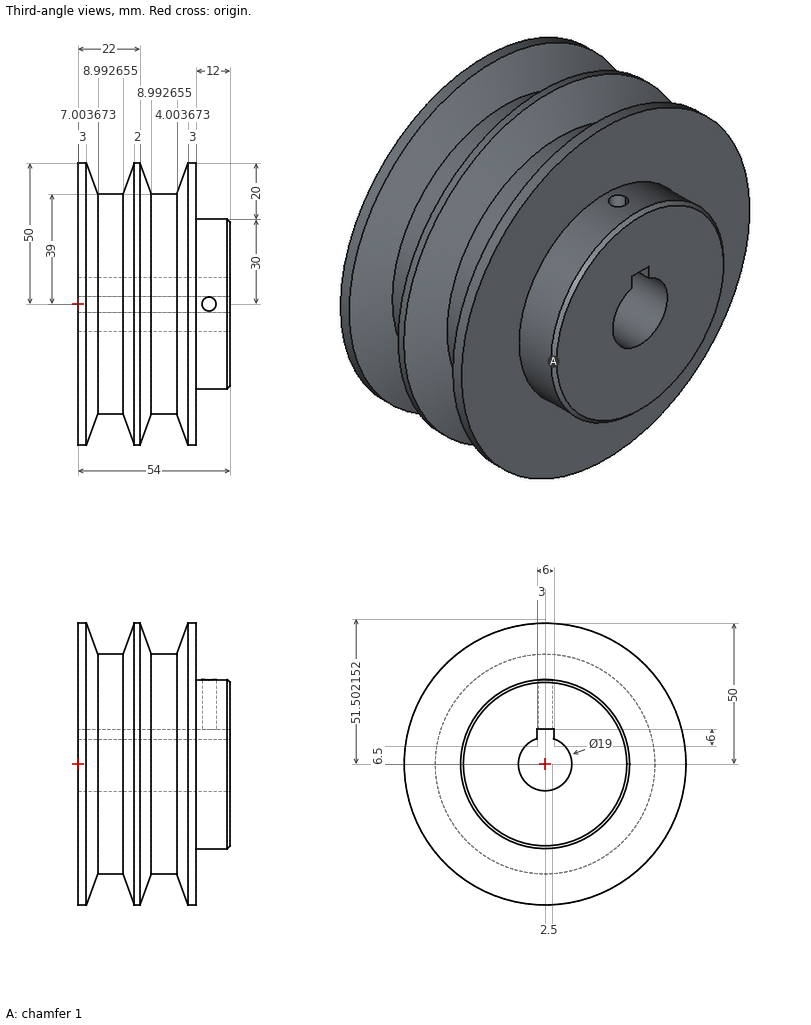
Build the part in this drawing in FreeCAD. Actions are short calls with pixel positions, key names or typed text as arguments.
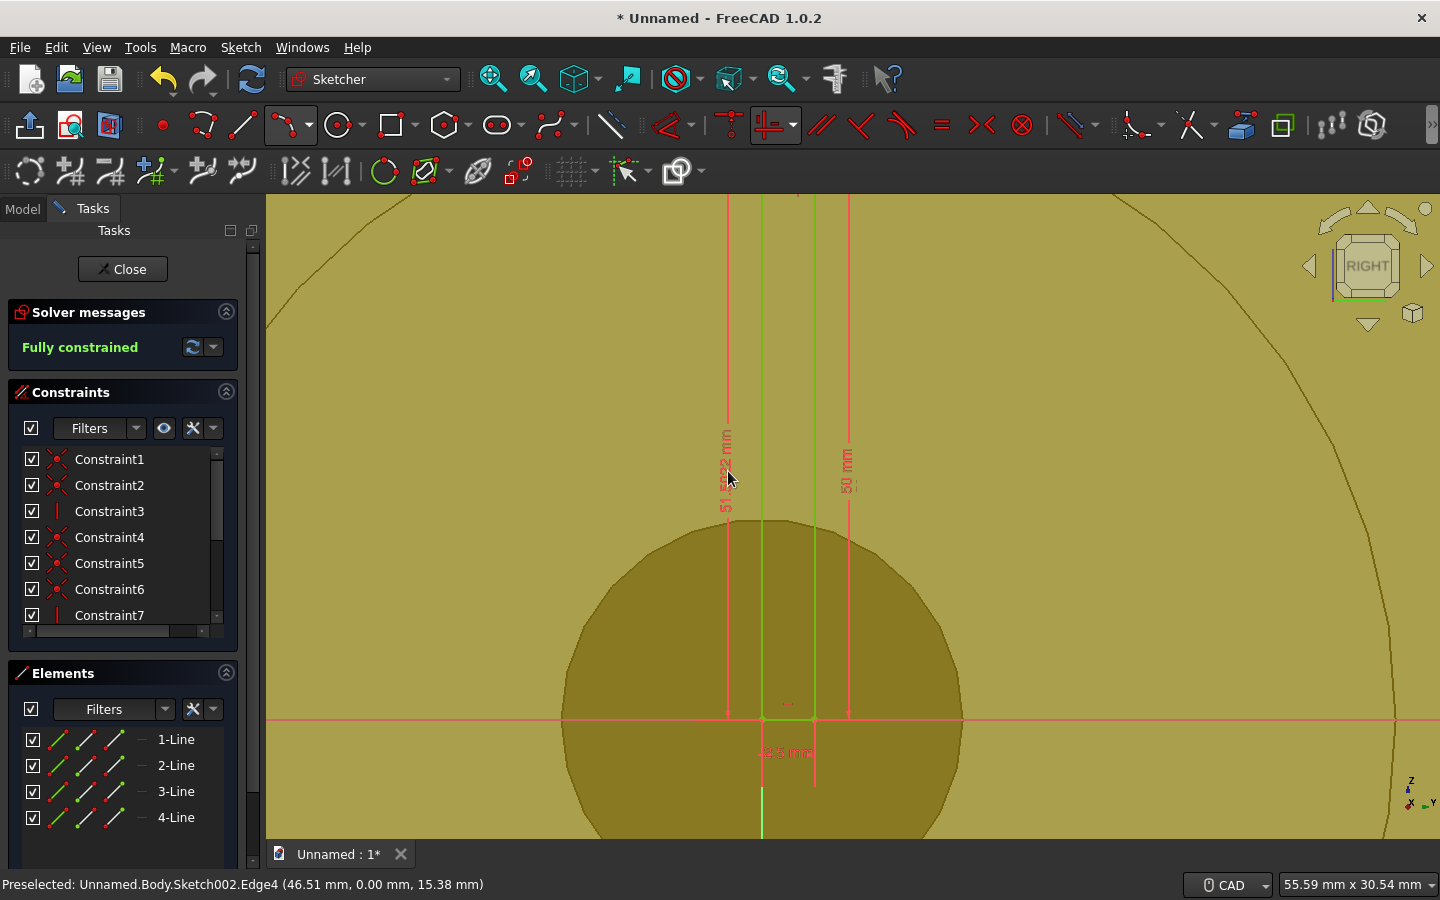
click(123, 269)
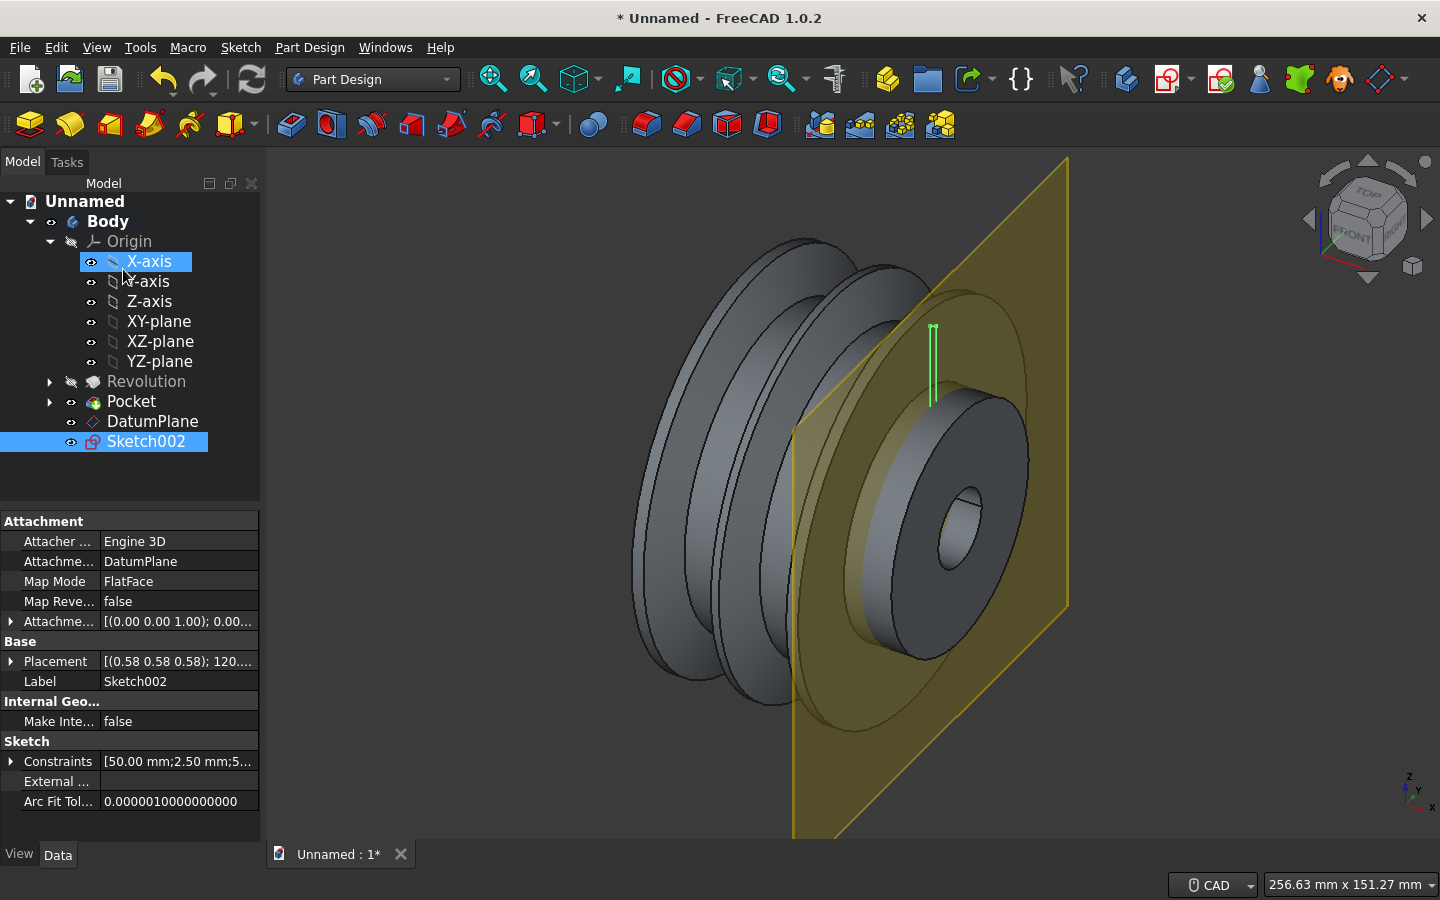
click(372, 124)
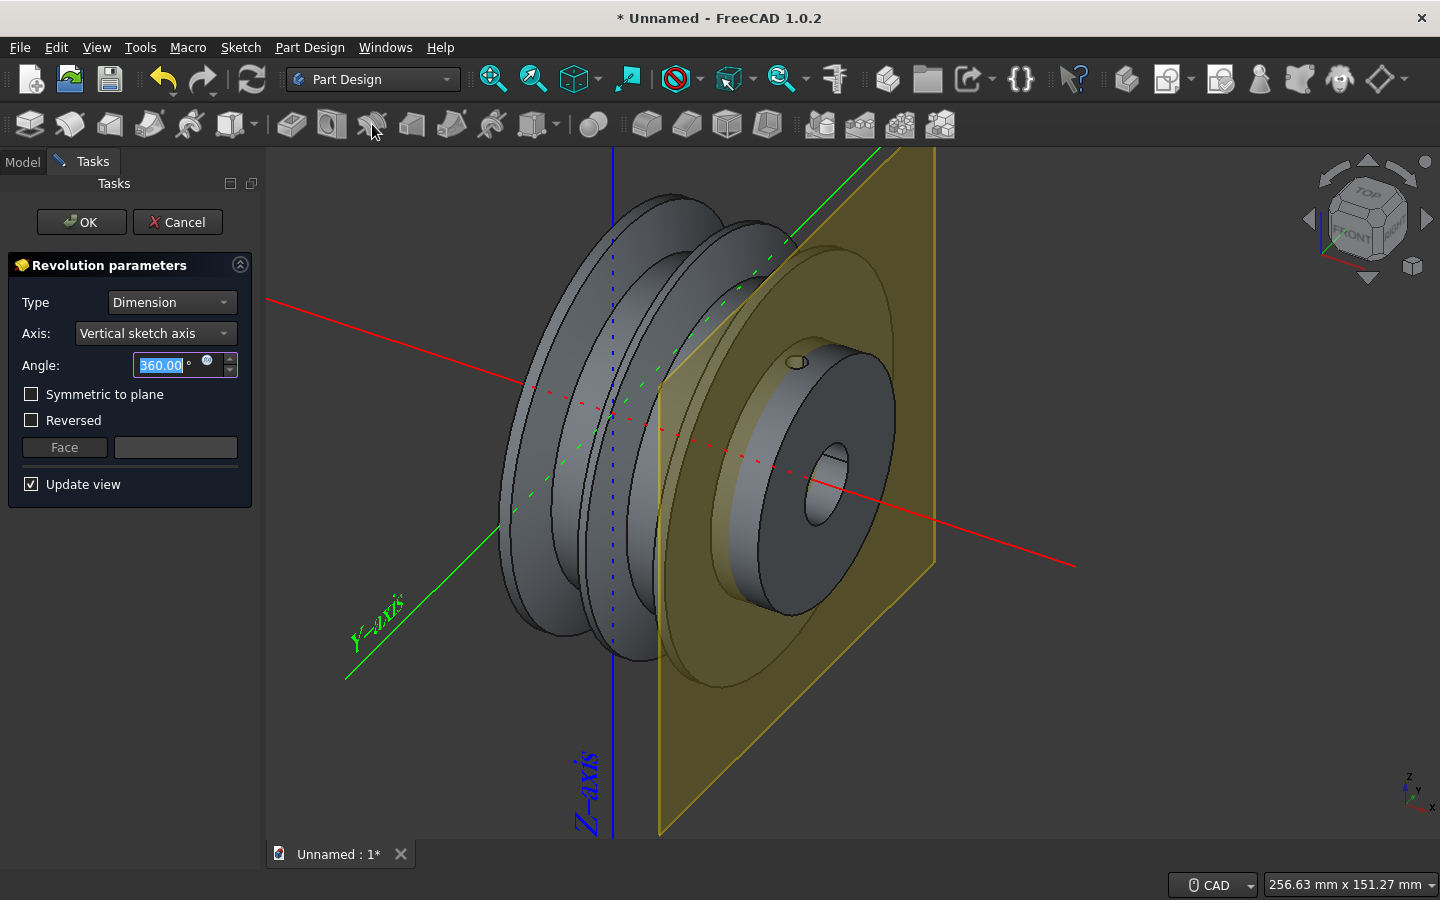
click(82, 222)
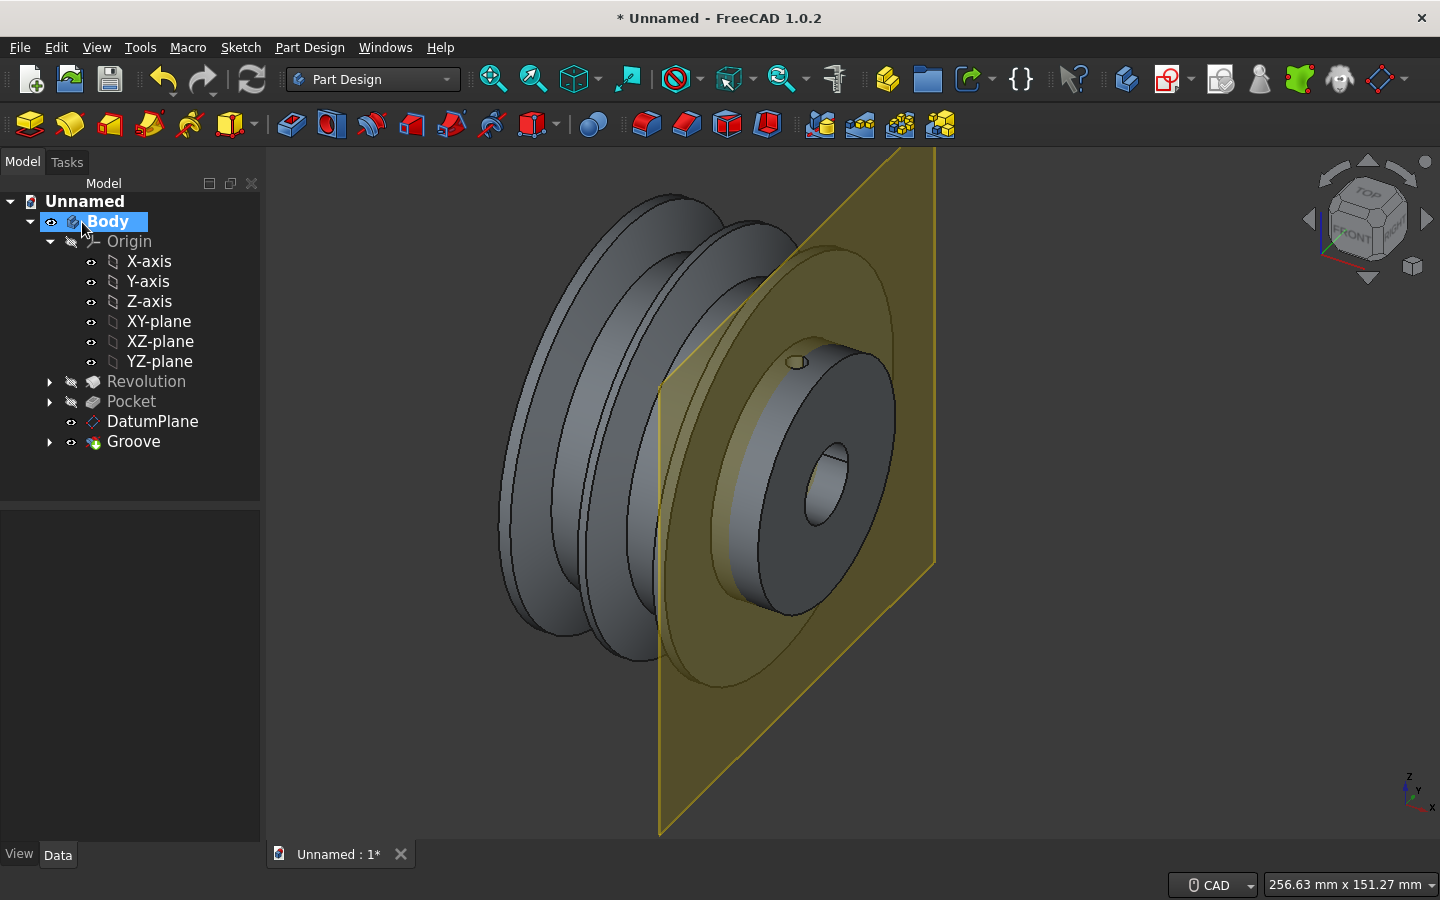
click(116, 422)
key(space)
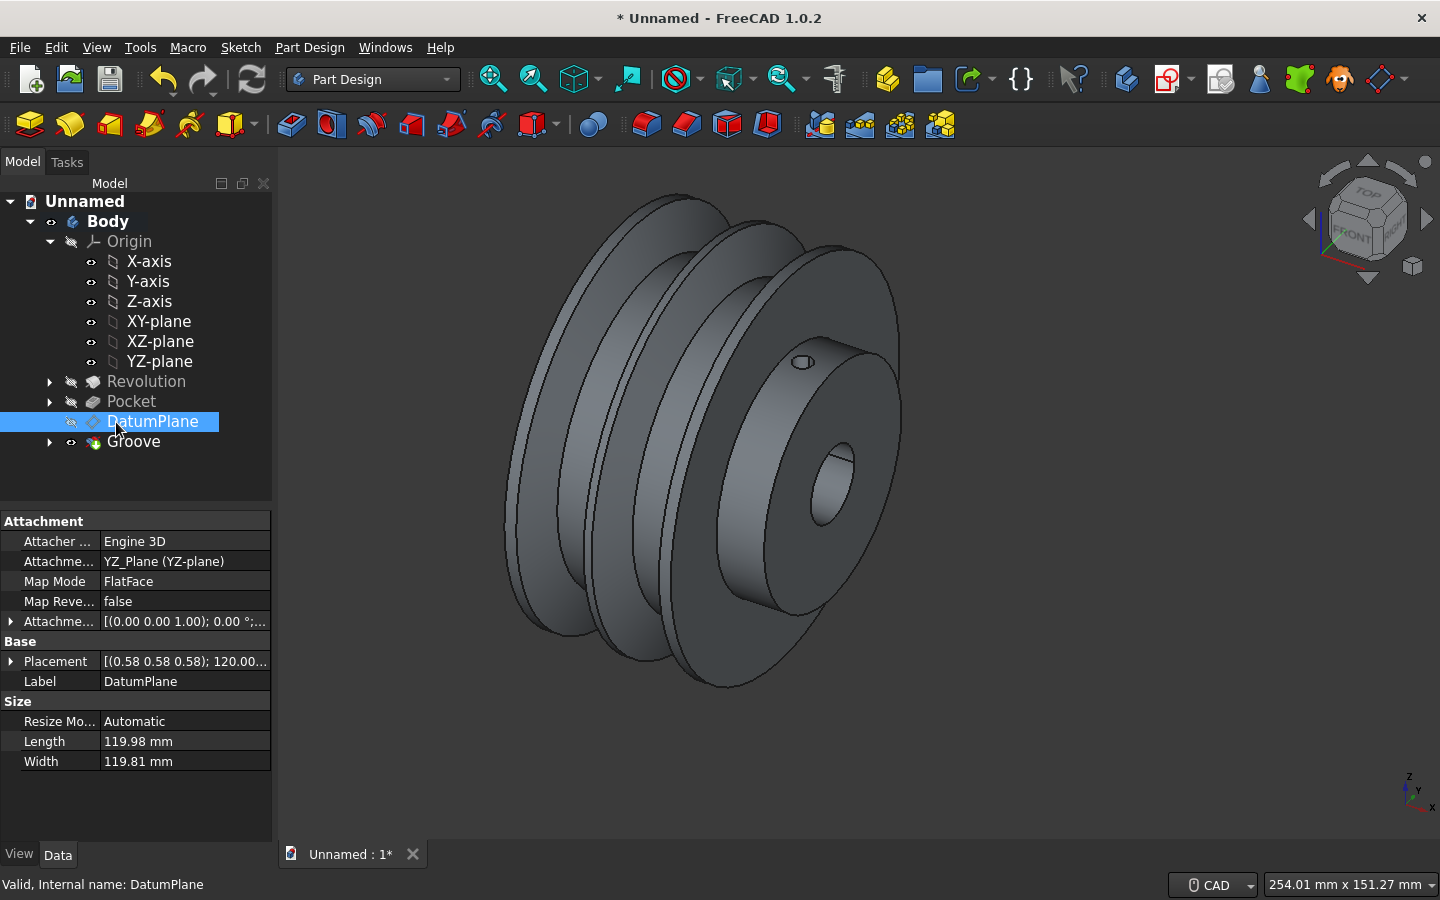
click(494, 80)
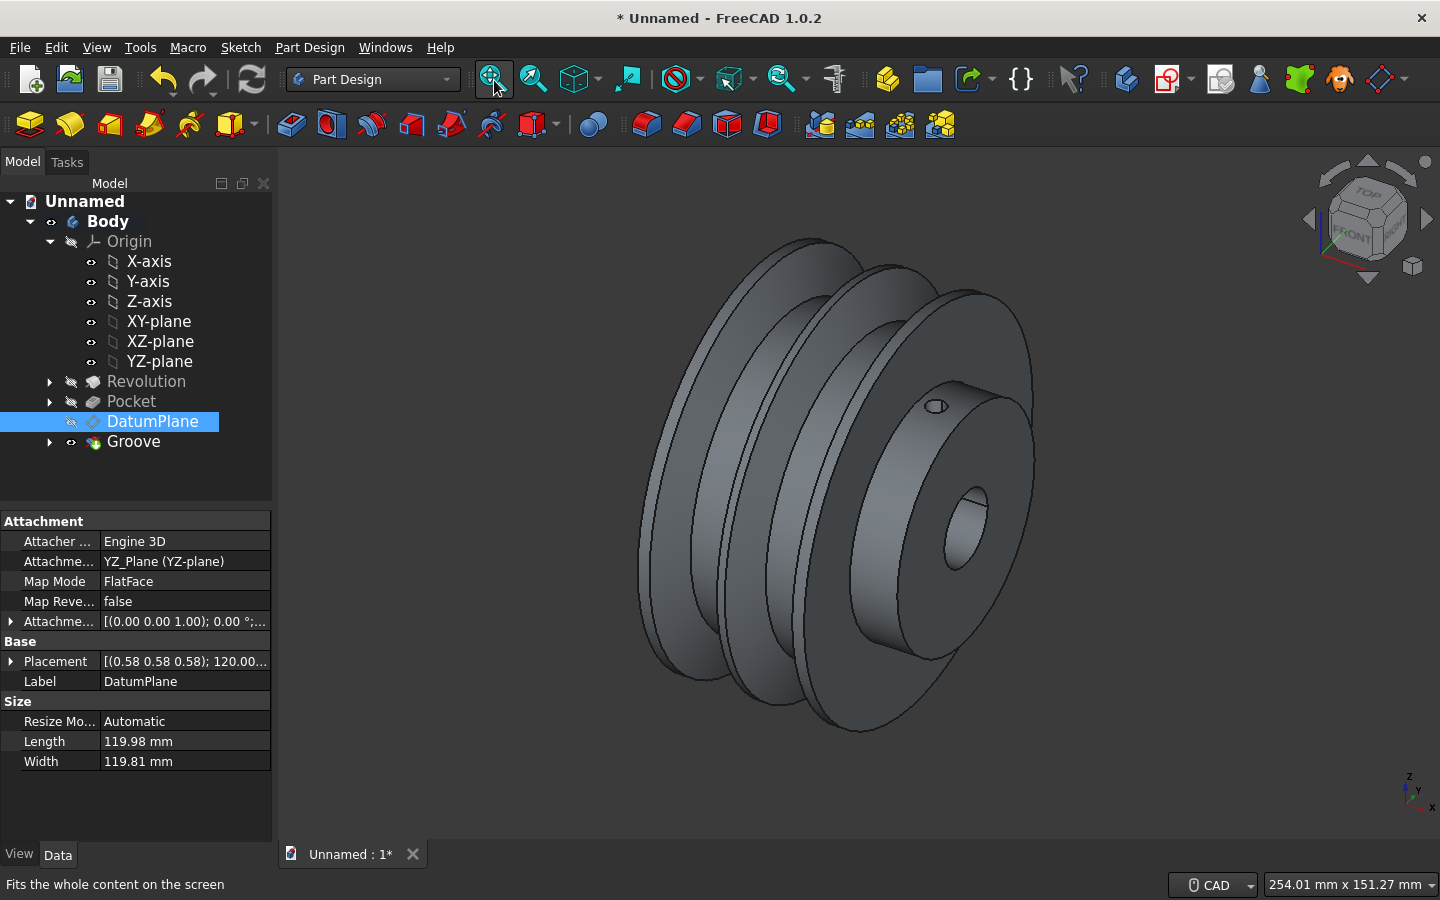
click(897, 596)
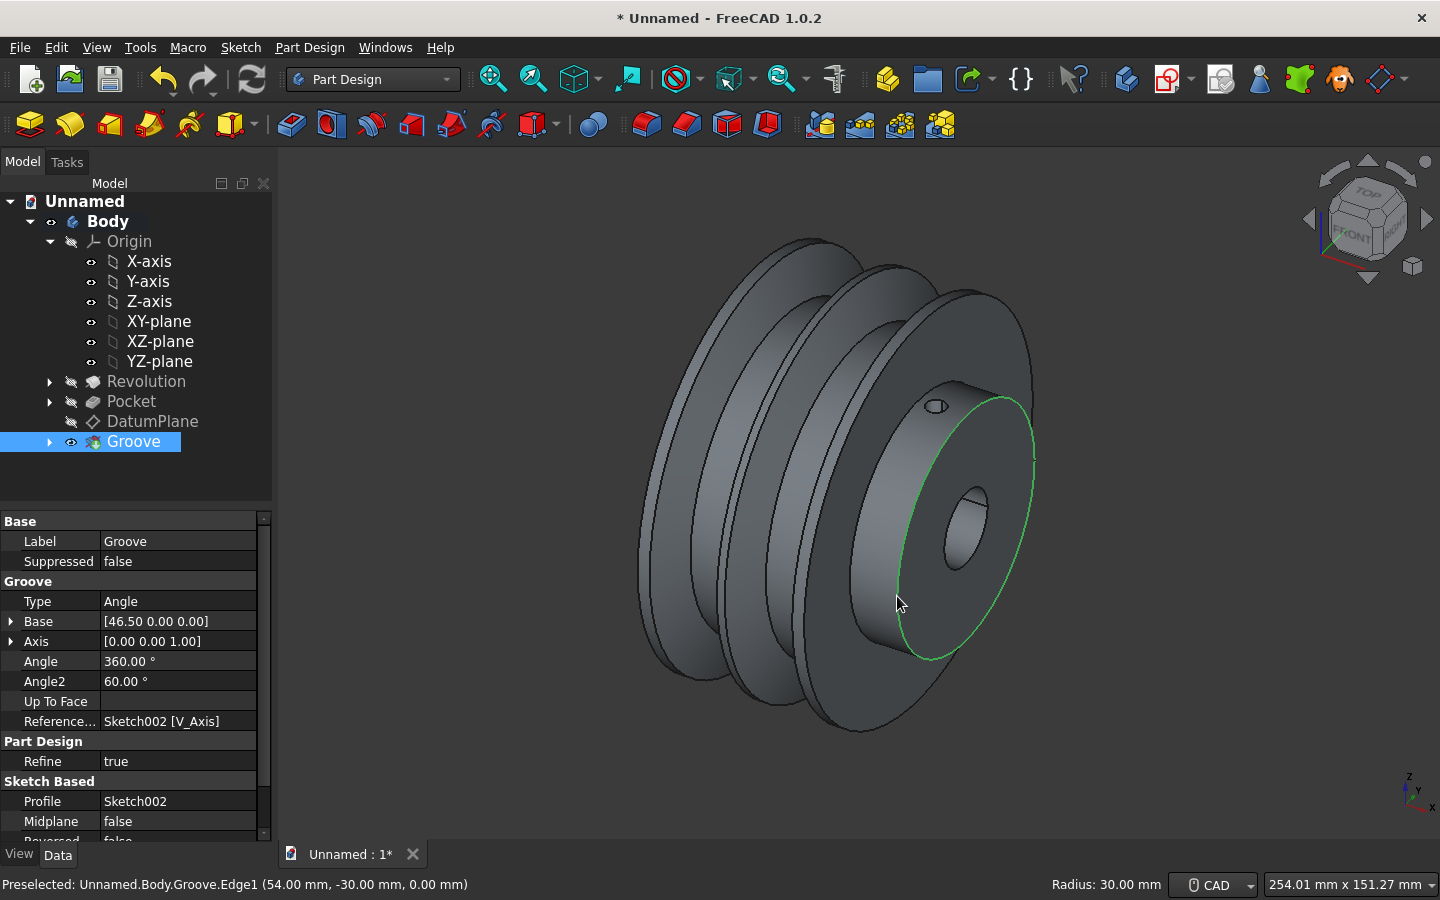
click(688, 124)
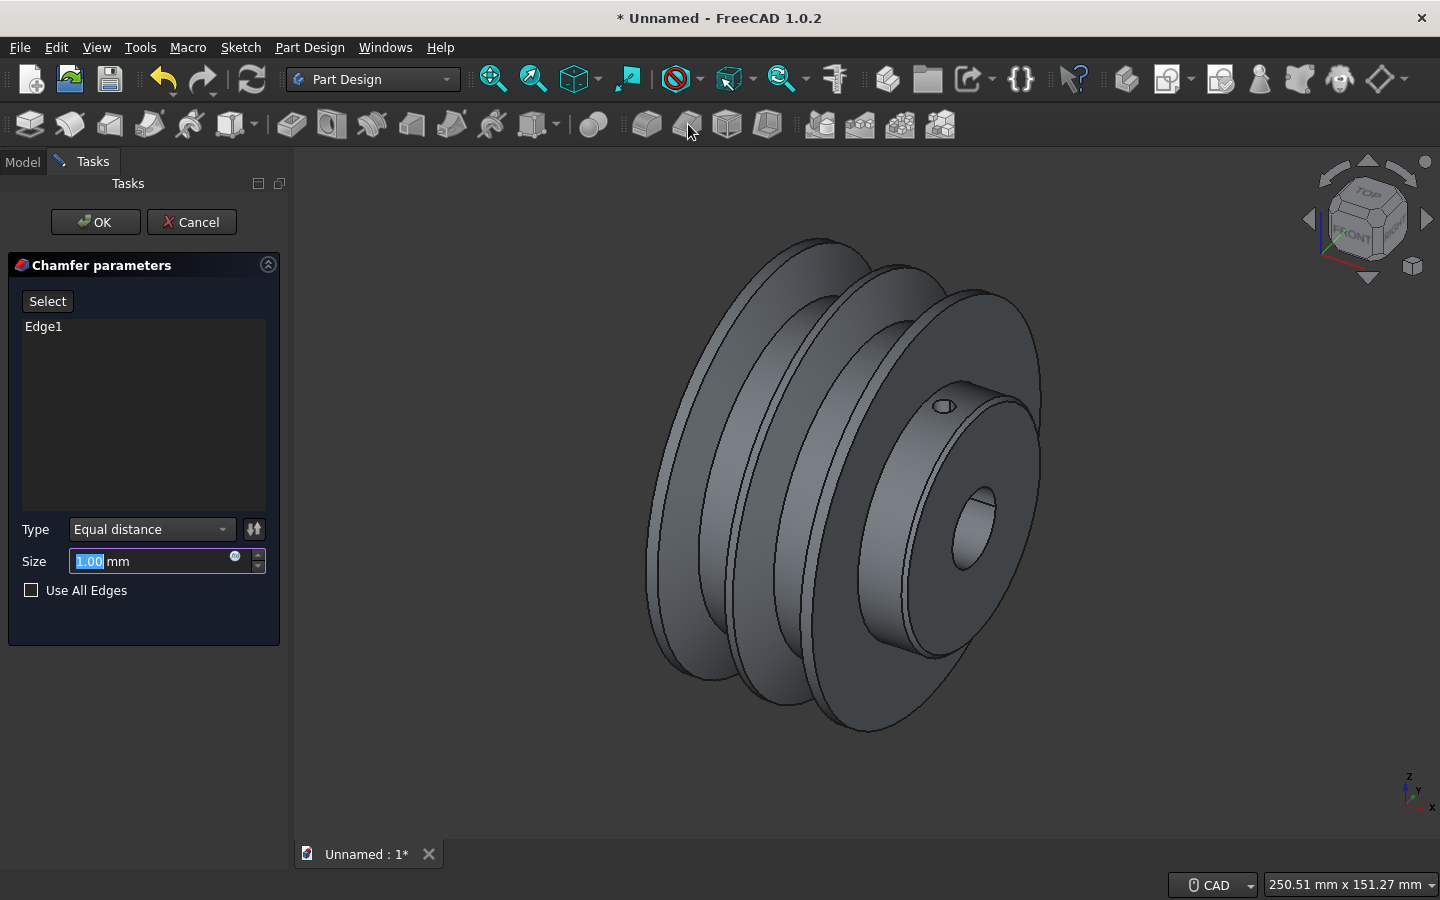
text(1)
key(Tab)